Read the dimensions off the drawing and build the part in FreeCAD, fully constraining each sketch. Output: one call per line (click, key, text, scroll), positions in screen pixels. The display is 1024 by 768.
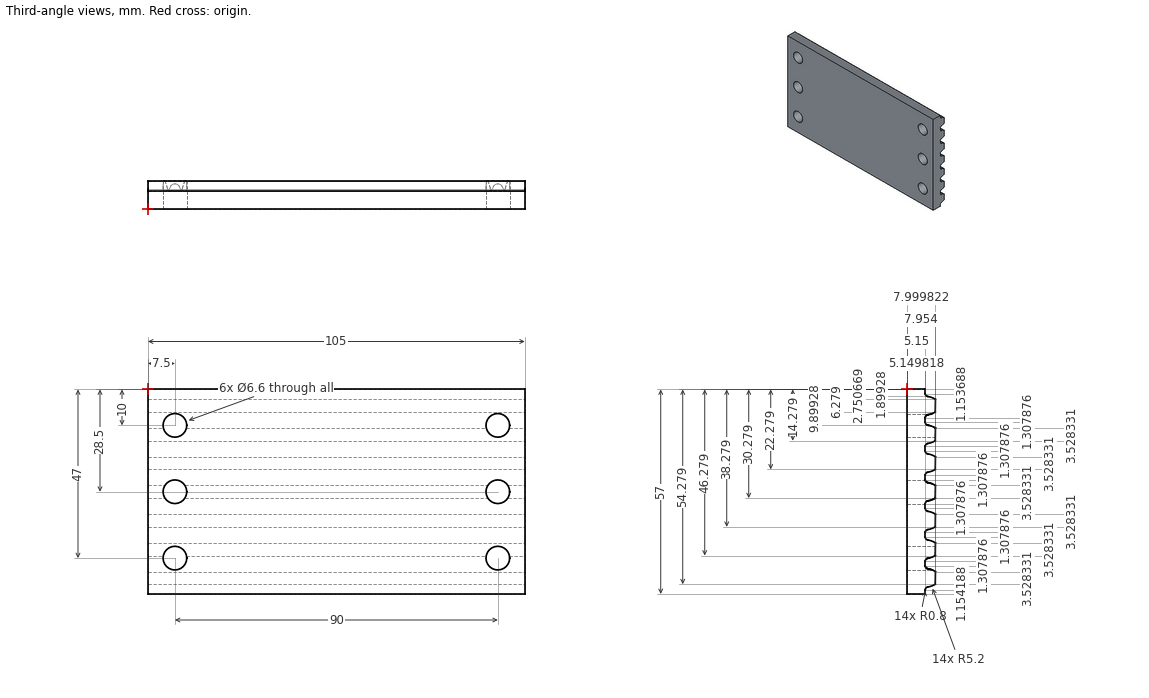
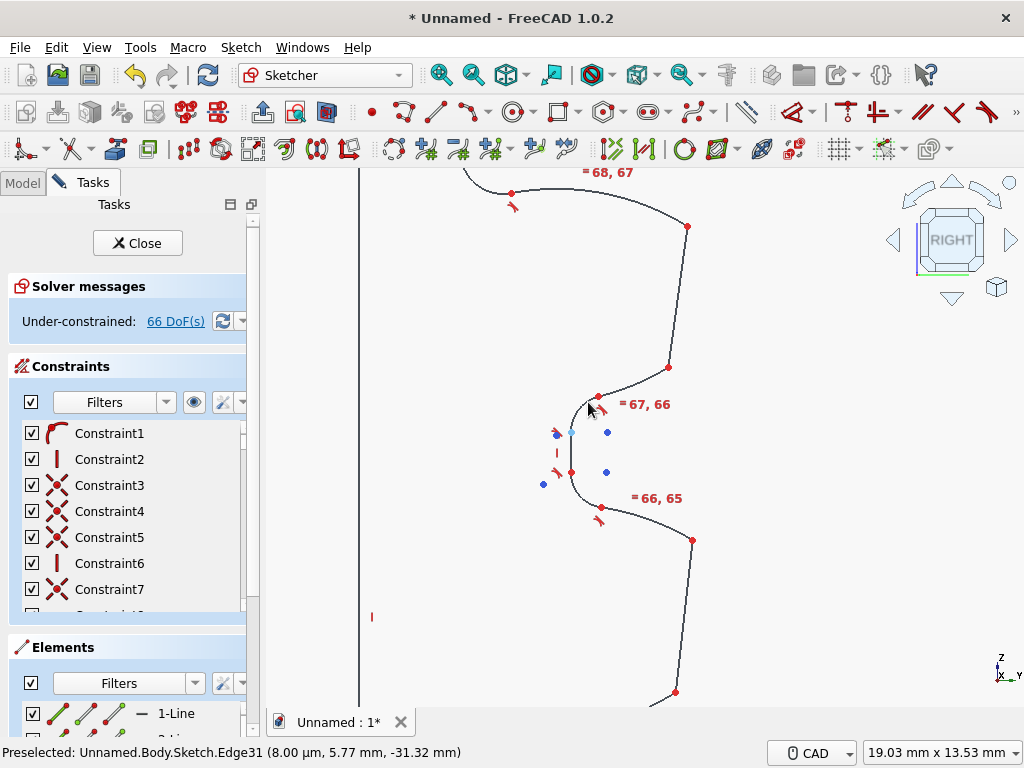
click(586, 403)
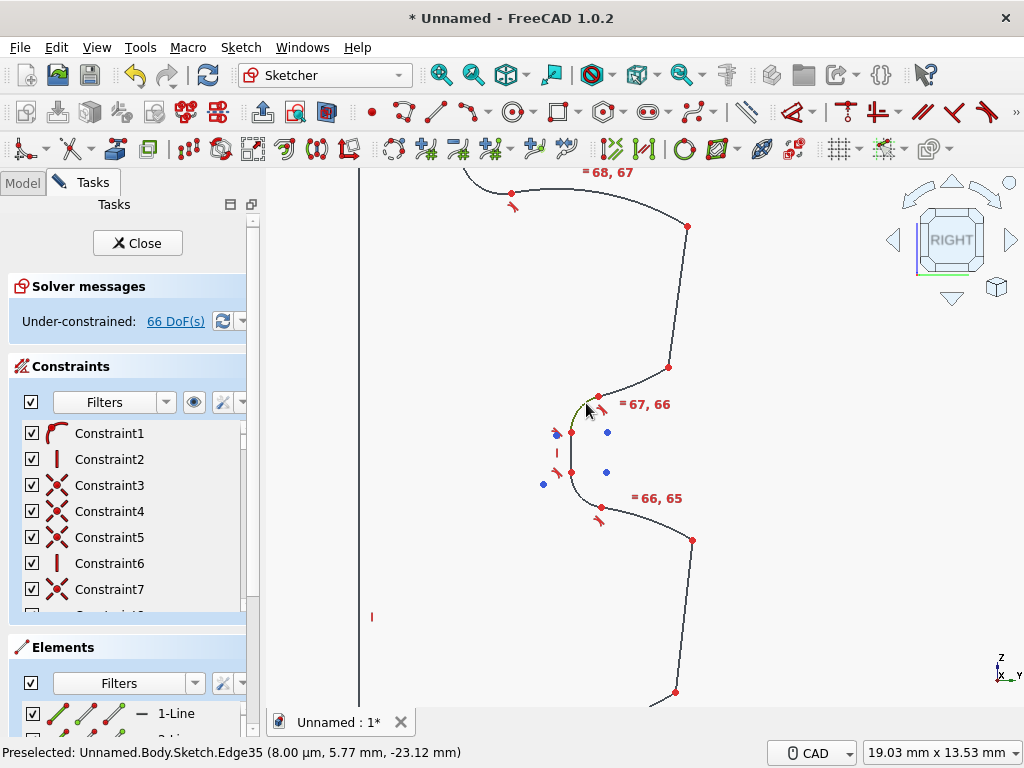
scroll(588, 402, down, 9)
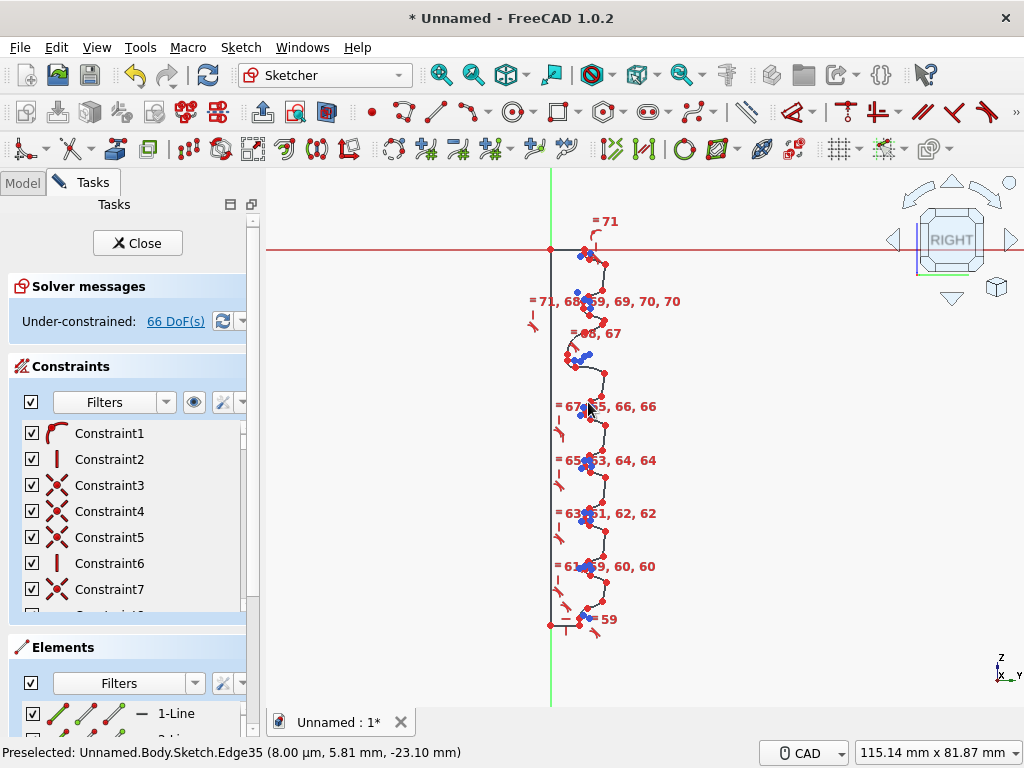
scroll(577, 336, up, 3)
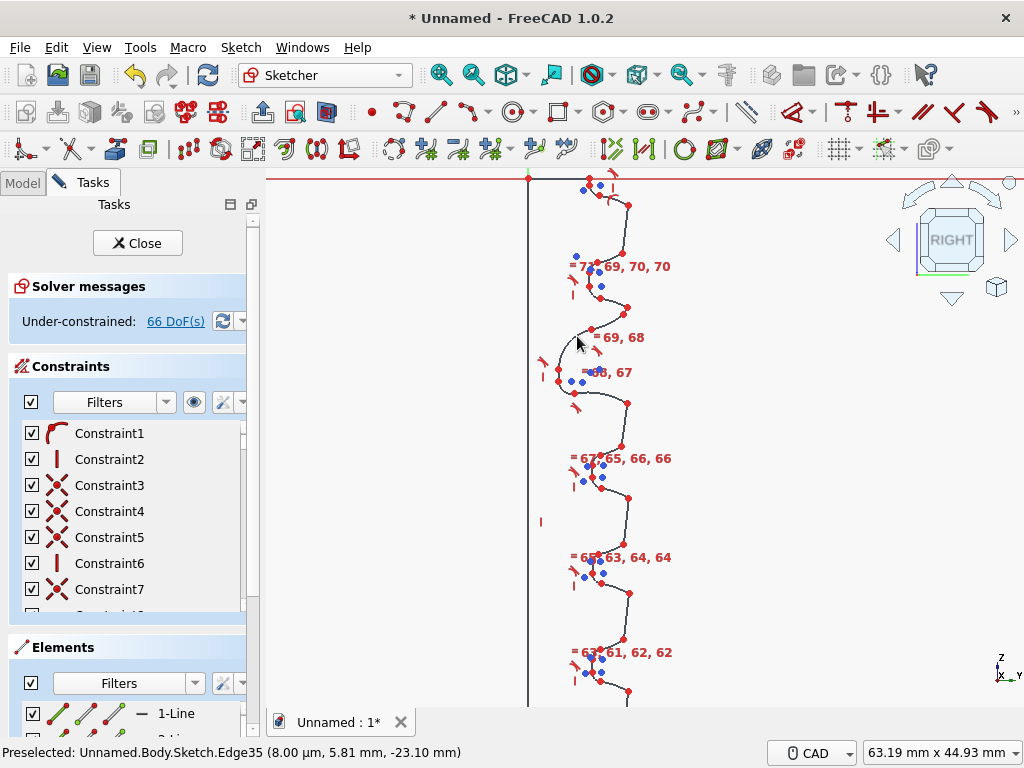
click(576, 336)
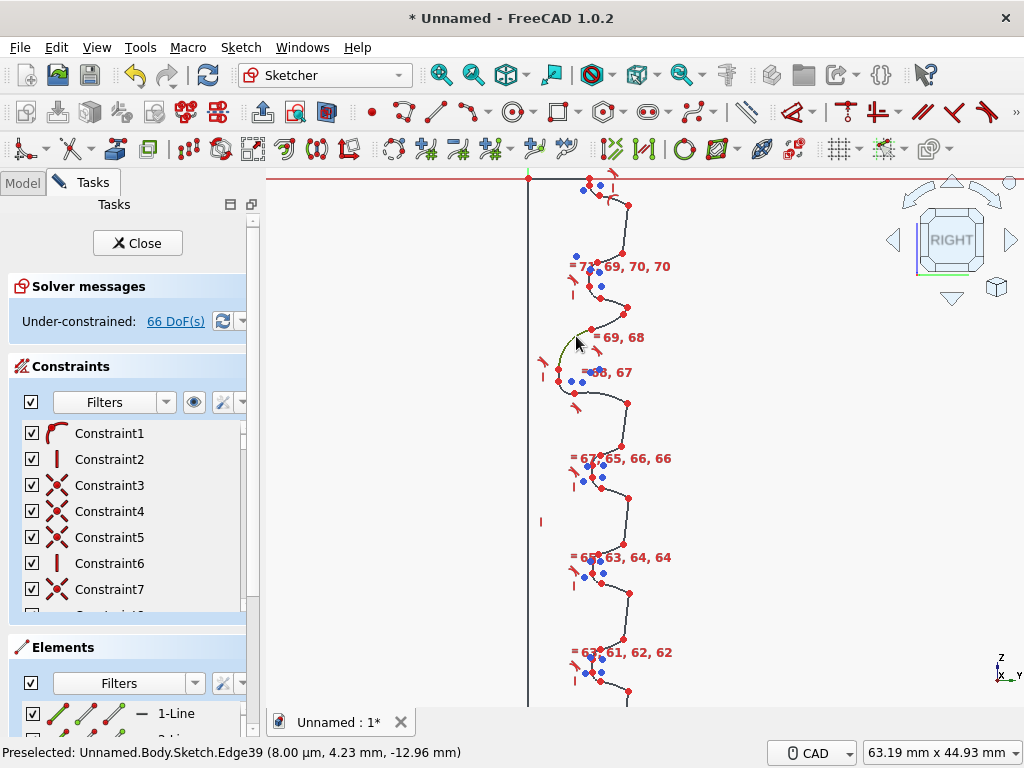
scroll(592, 266, up, 4)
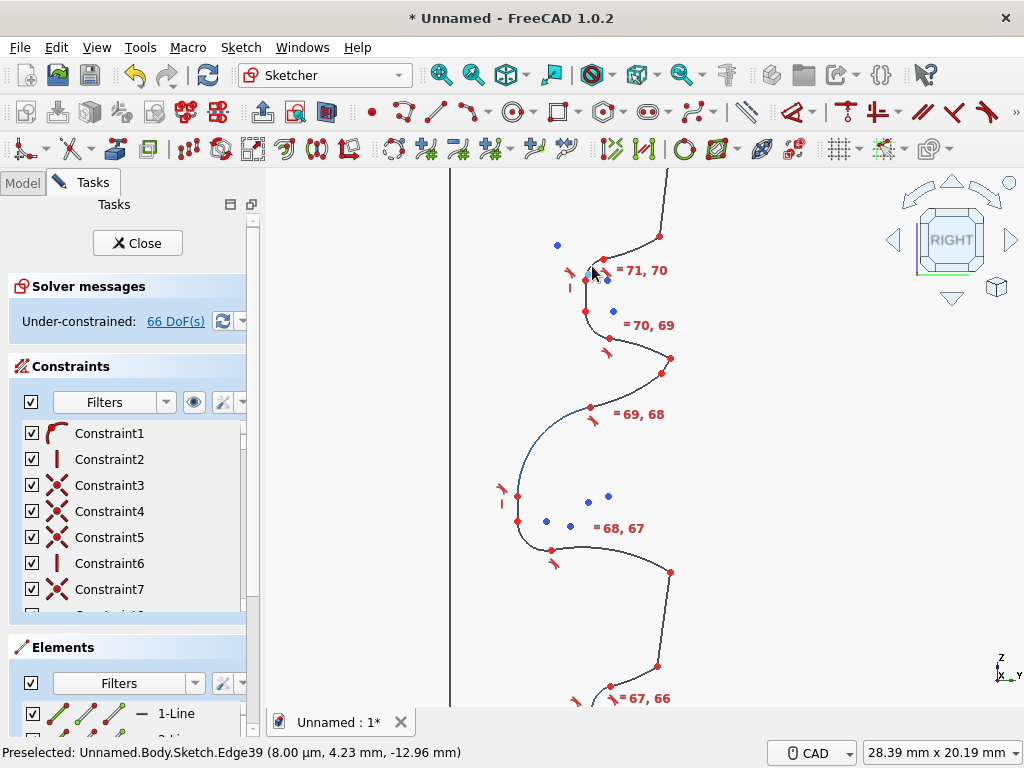
click(591, 267)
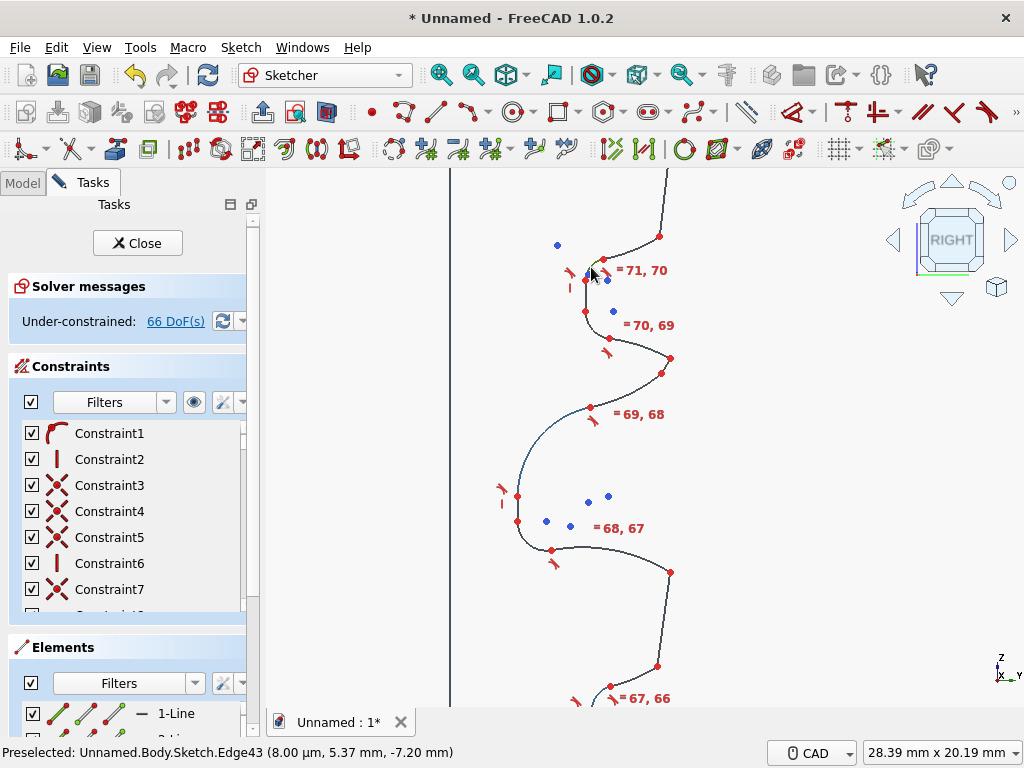
key(e)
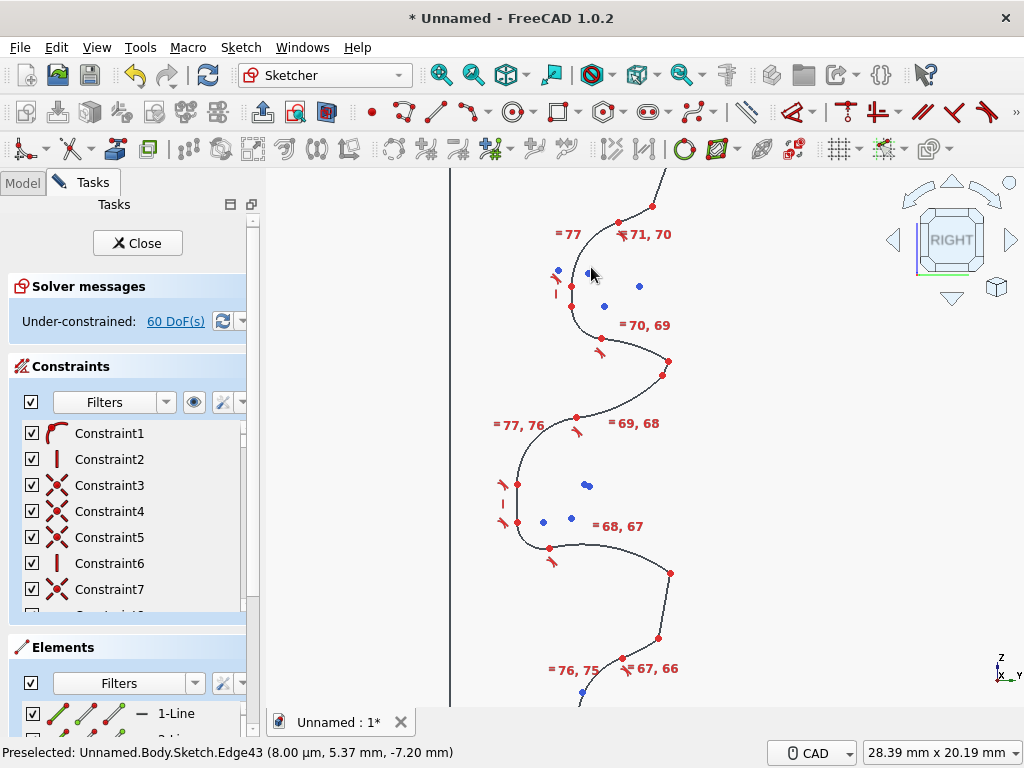
scroll(583, 308, down, 7)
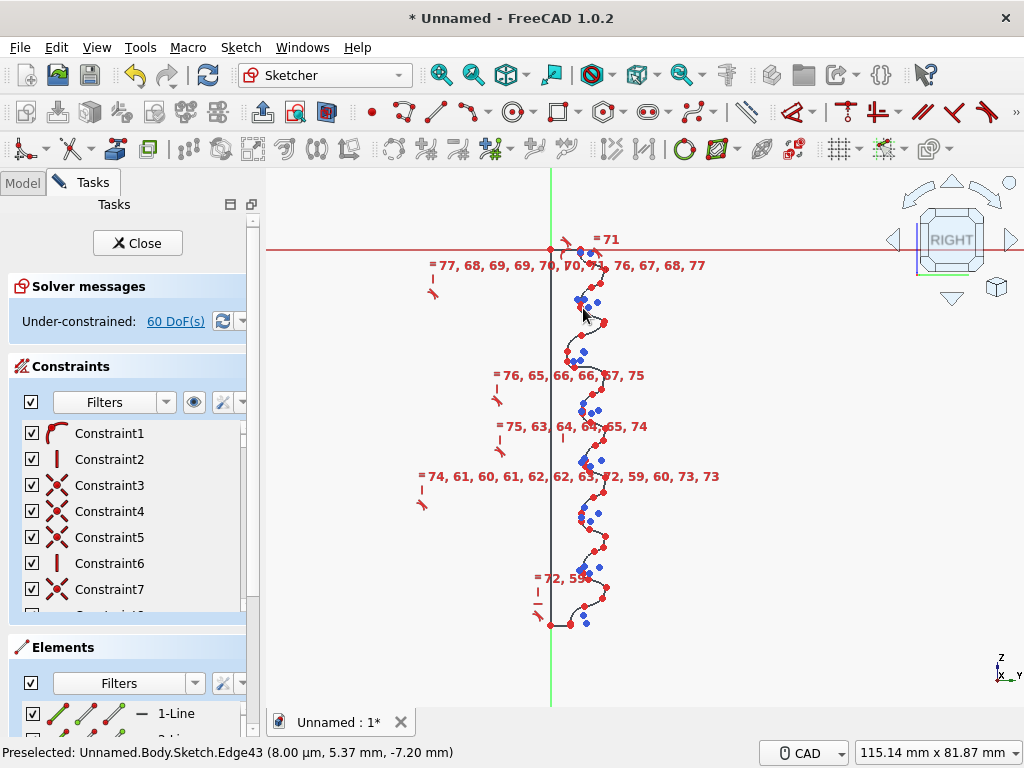
scroll(584, 576, up, 9)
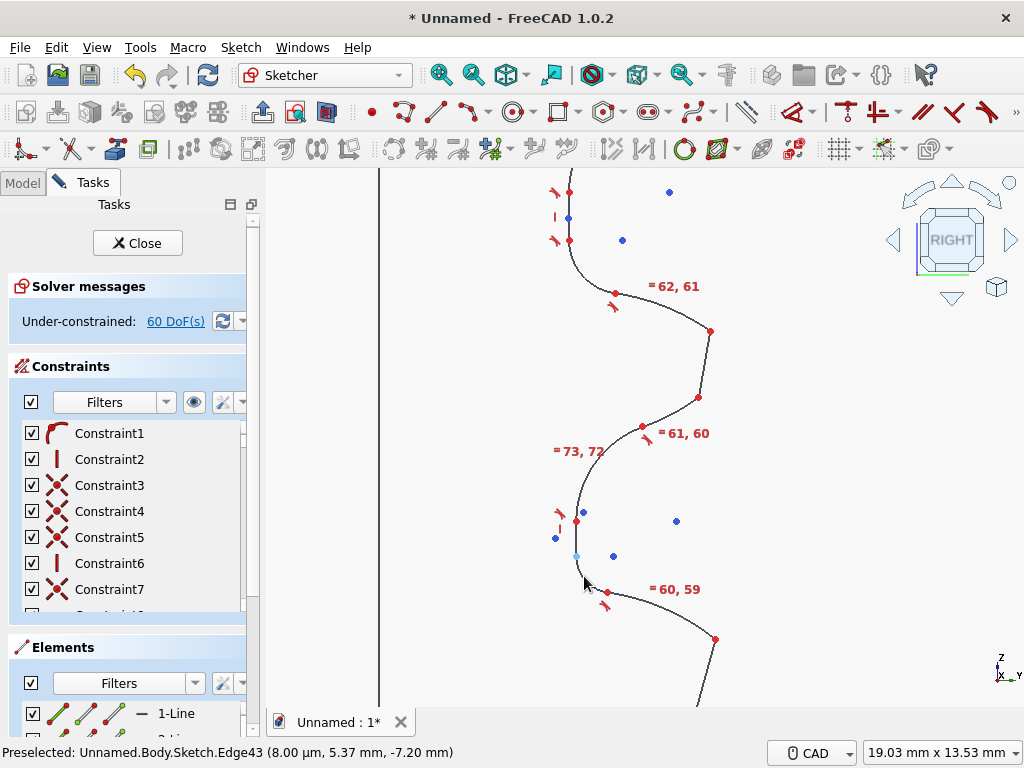
click(580, 572)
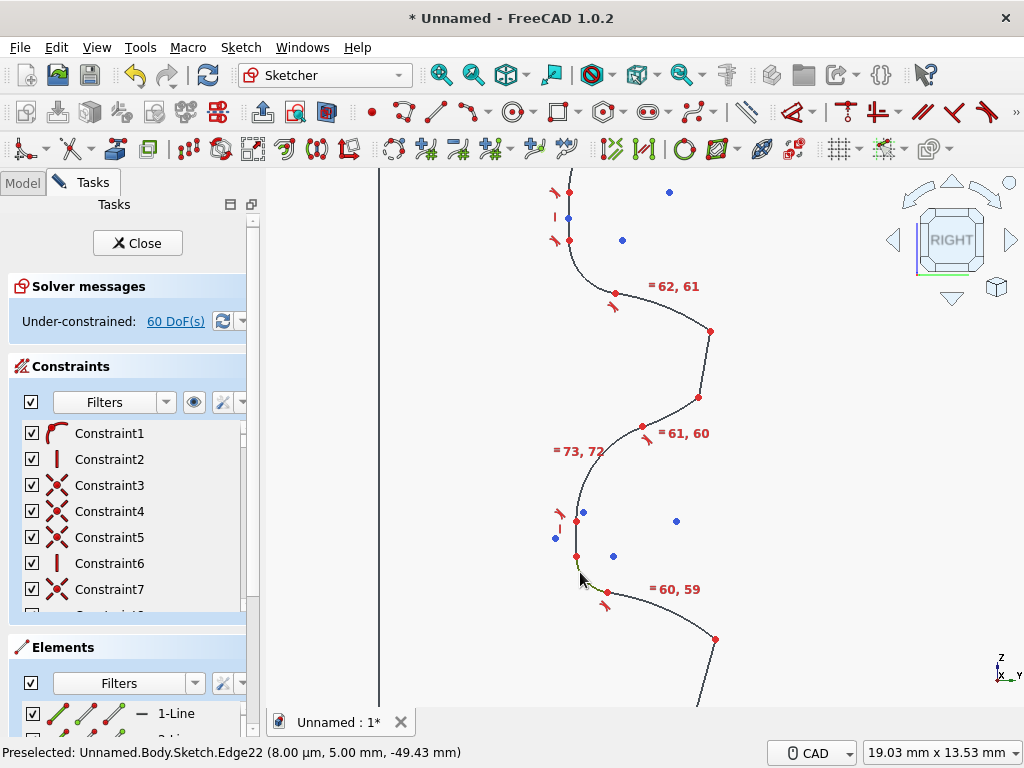
click(574, 262)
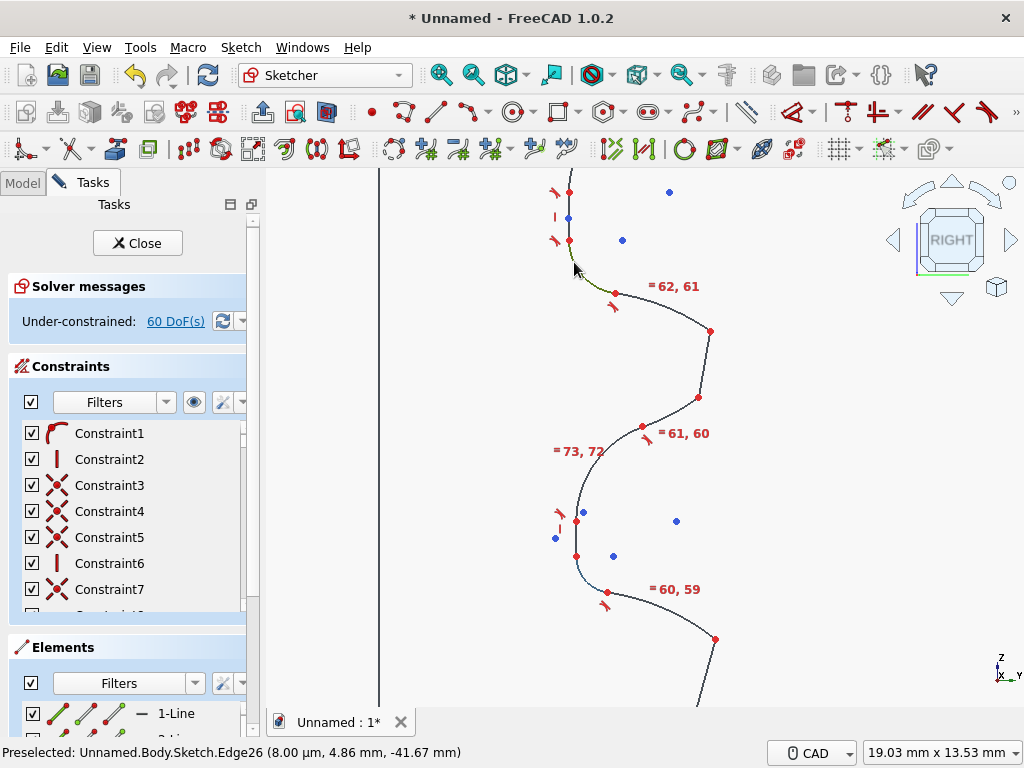
scroll(584, 577, down, 9)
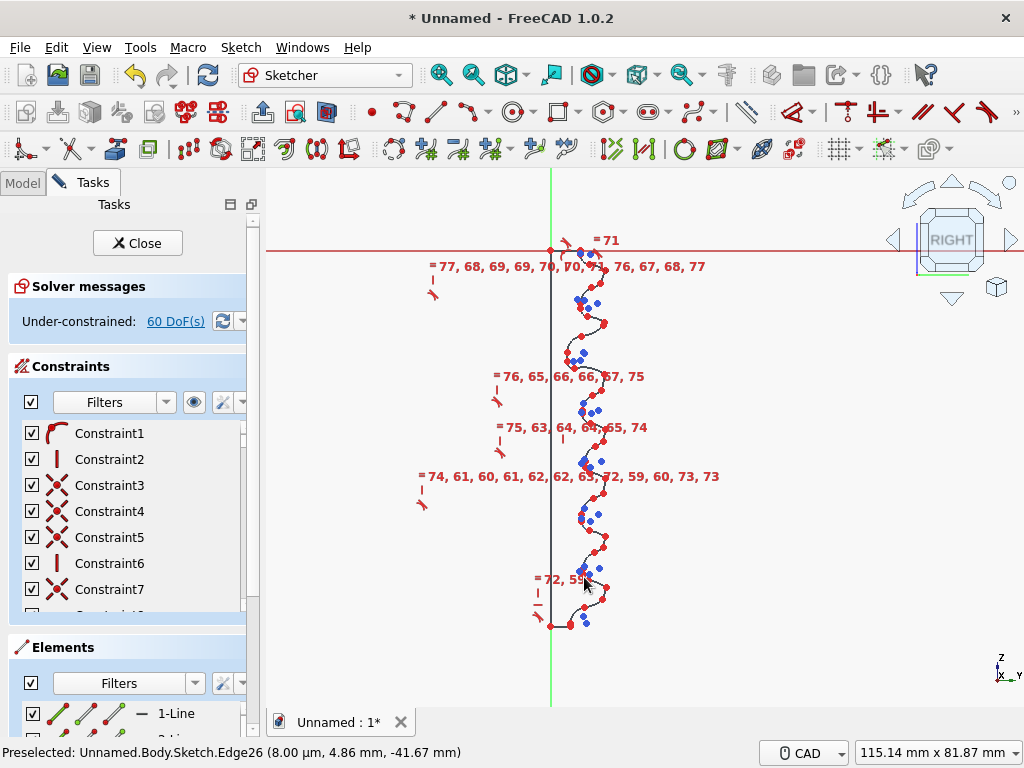
scroll(586, 470, up, 10)